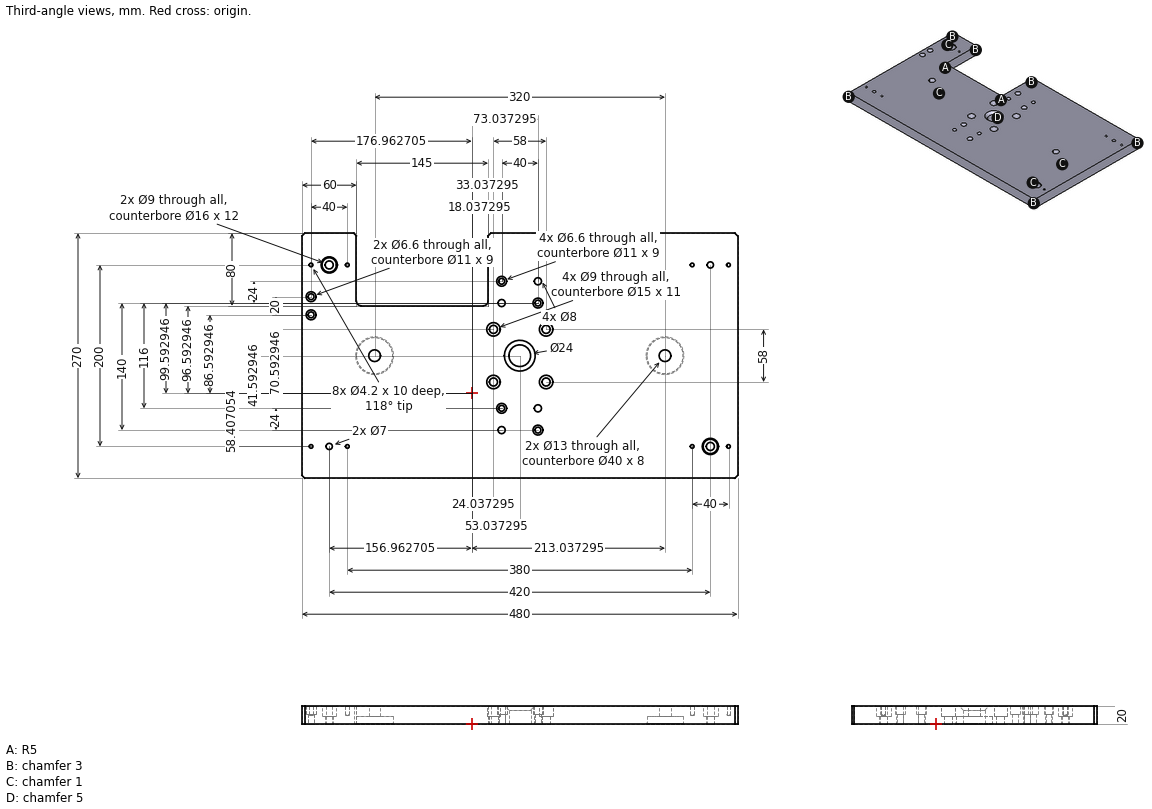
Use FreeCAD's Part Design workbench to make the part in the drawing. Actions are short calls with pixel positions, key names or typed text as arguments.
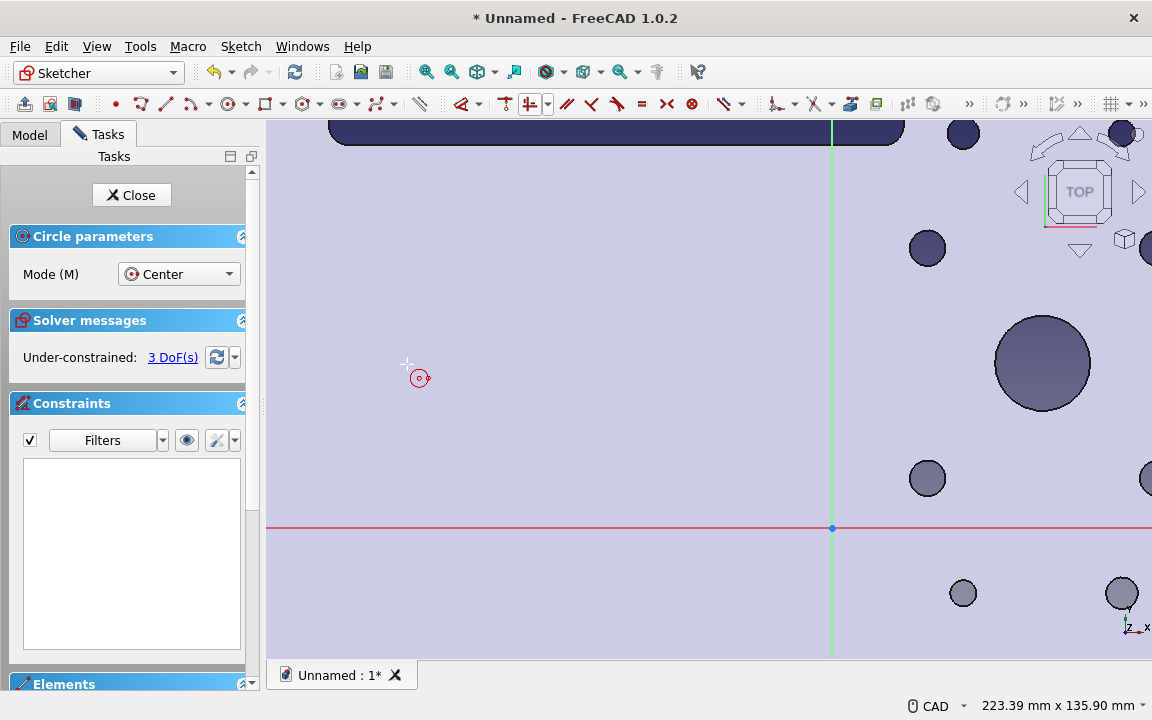
click(408, 363)
click(426, 345)
key(Escape)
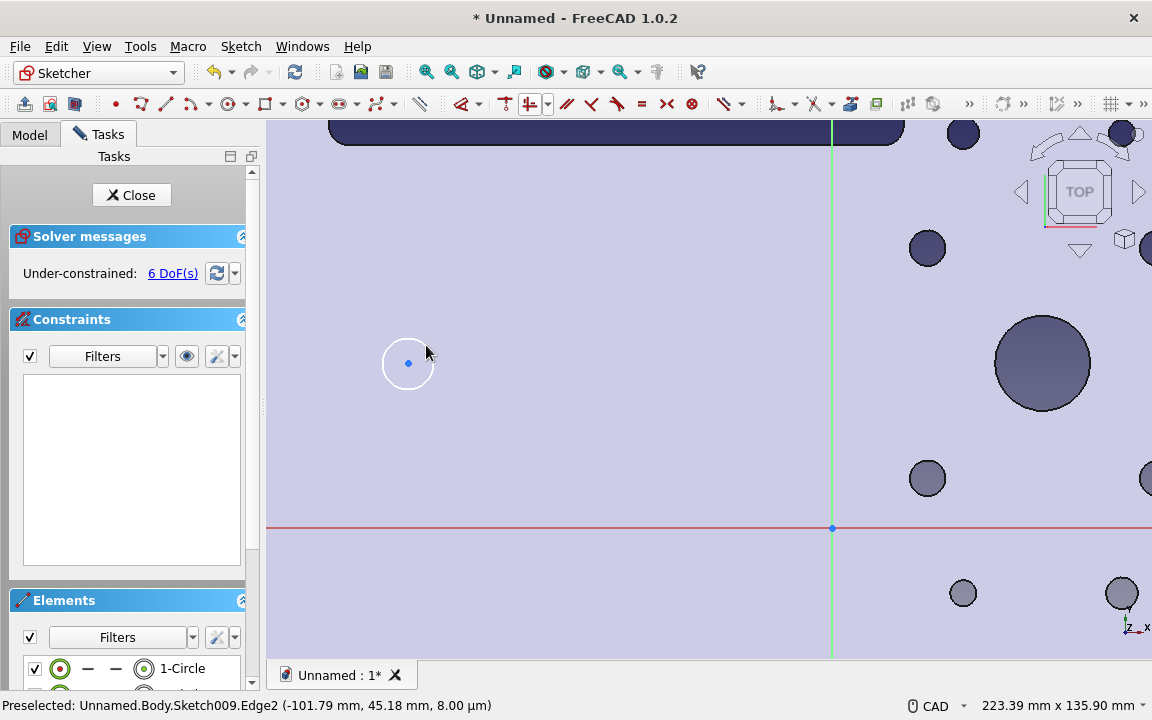
scroll(406, 364, down, 5)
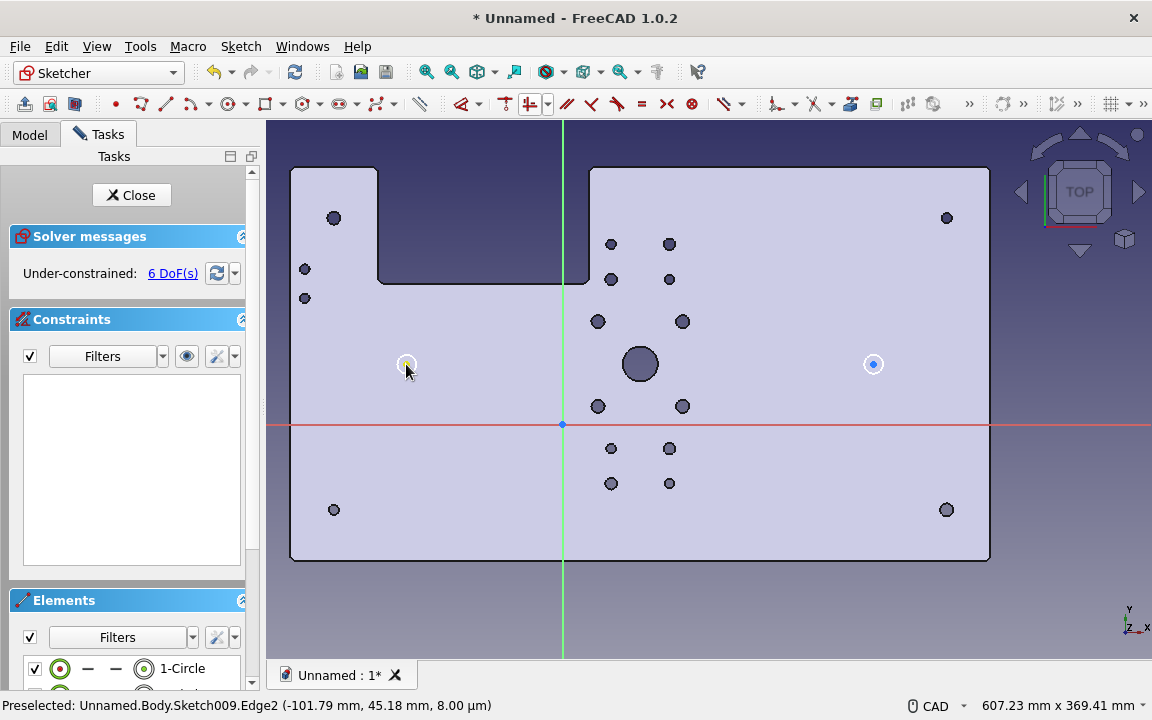
scroll(880, 358, up, 2)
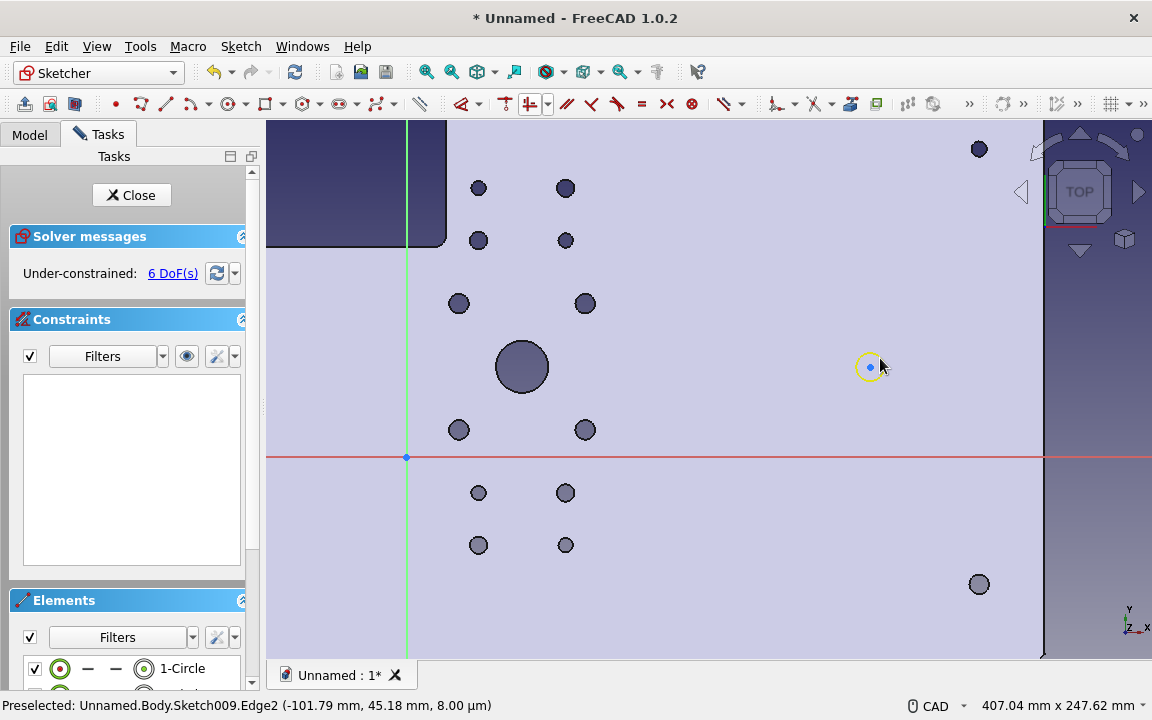
click(880, 357)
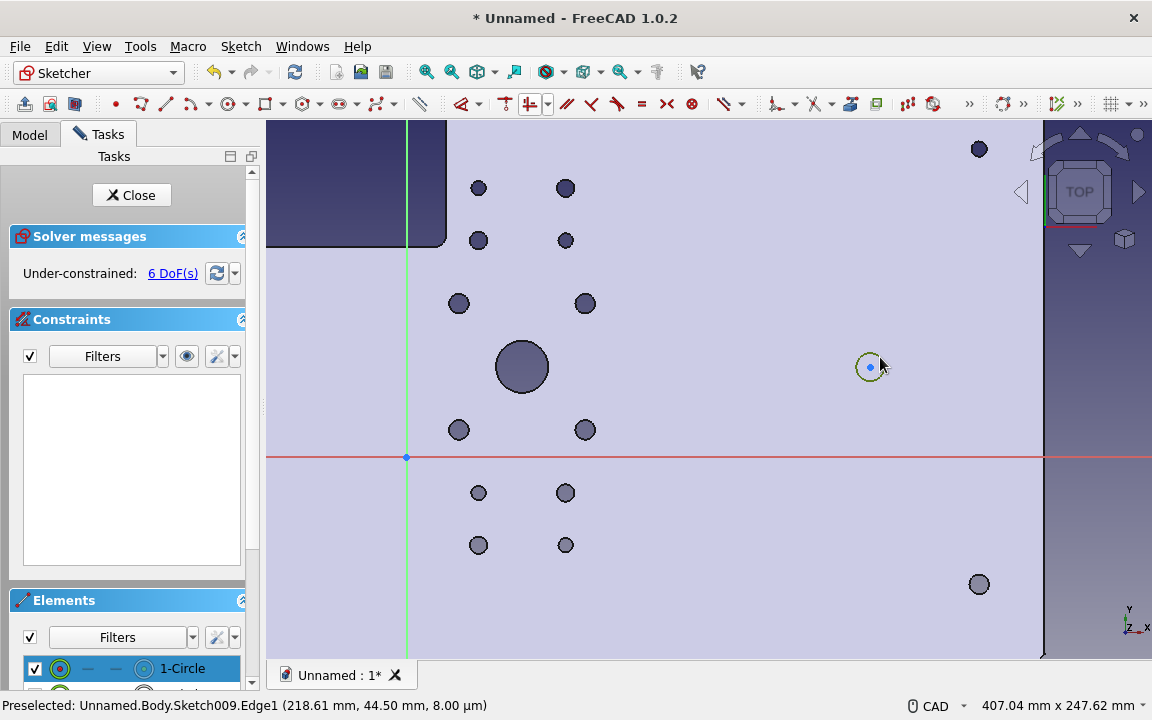
scroll(881, 358, down, 2)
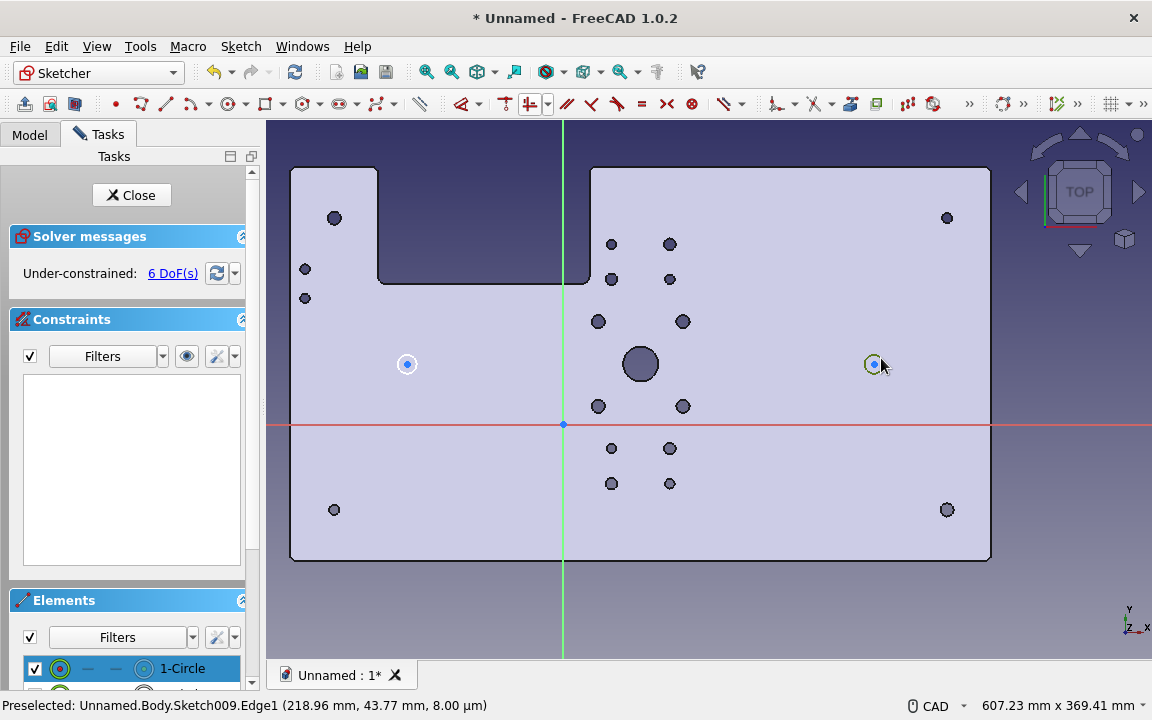
scroll(414, 358, up, 2)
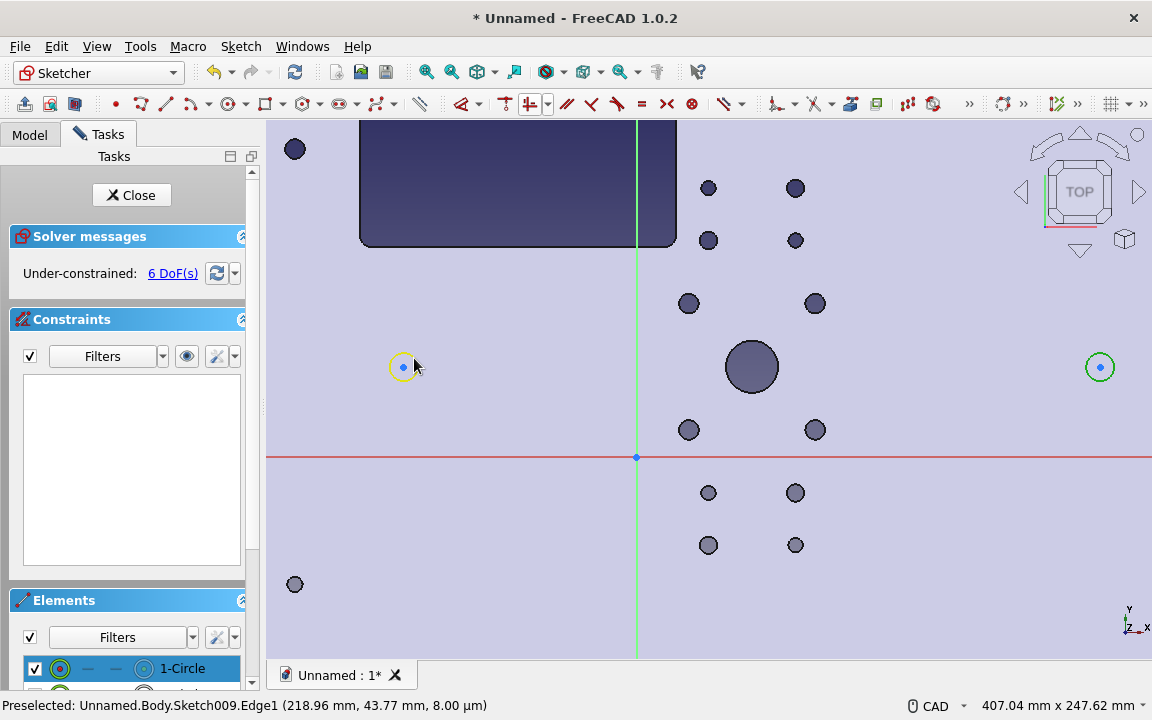
click(414, 357)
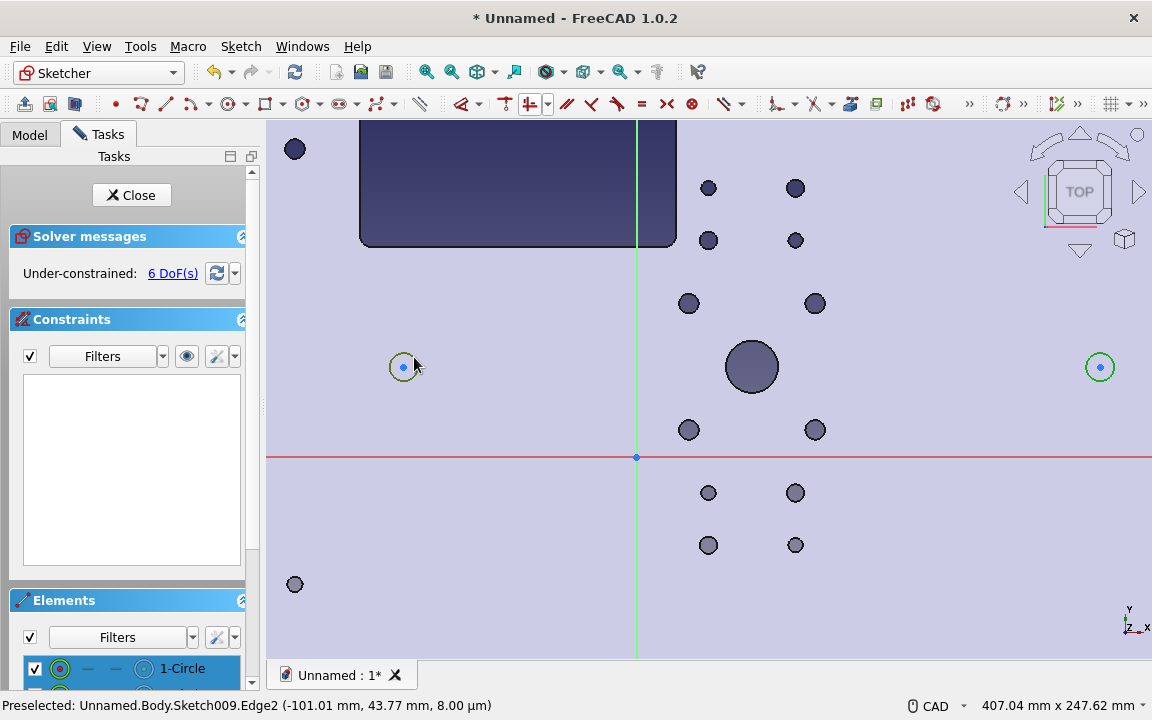
key(e)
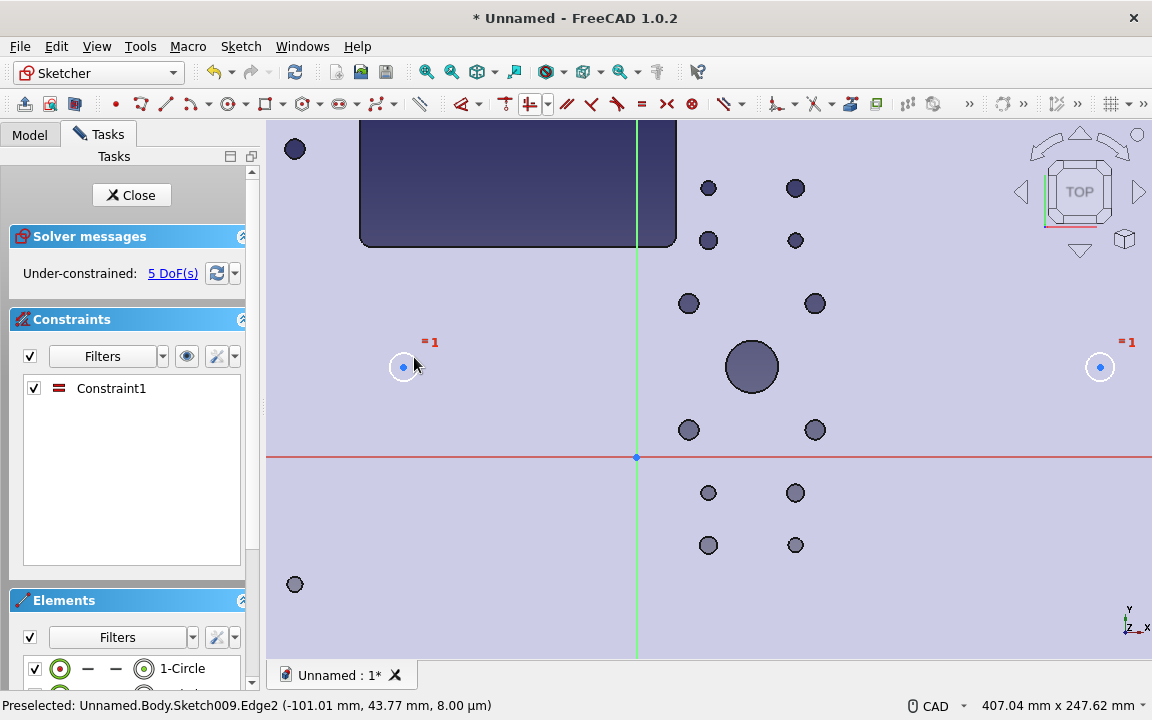
scroll(414, 358, down, 2)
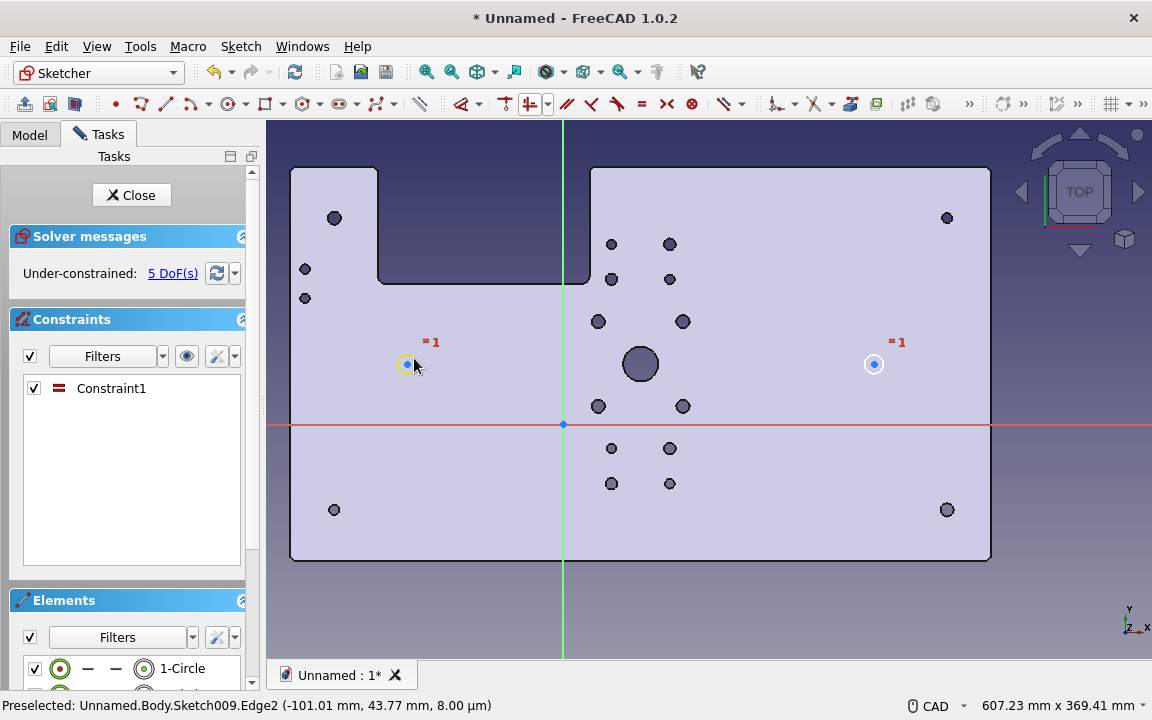
click(874, 364)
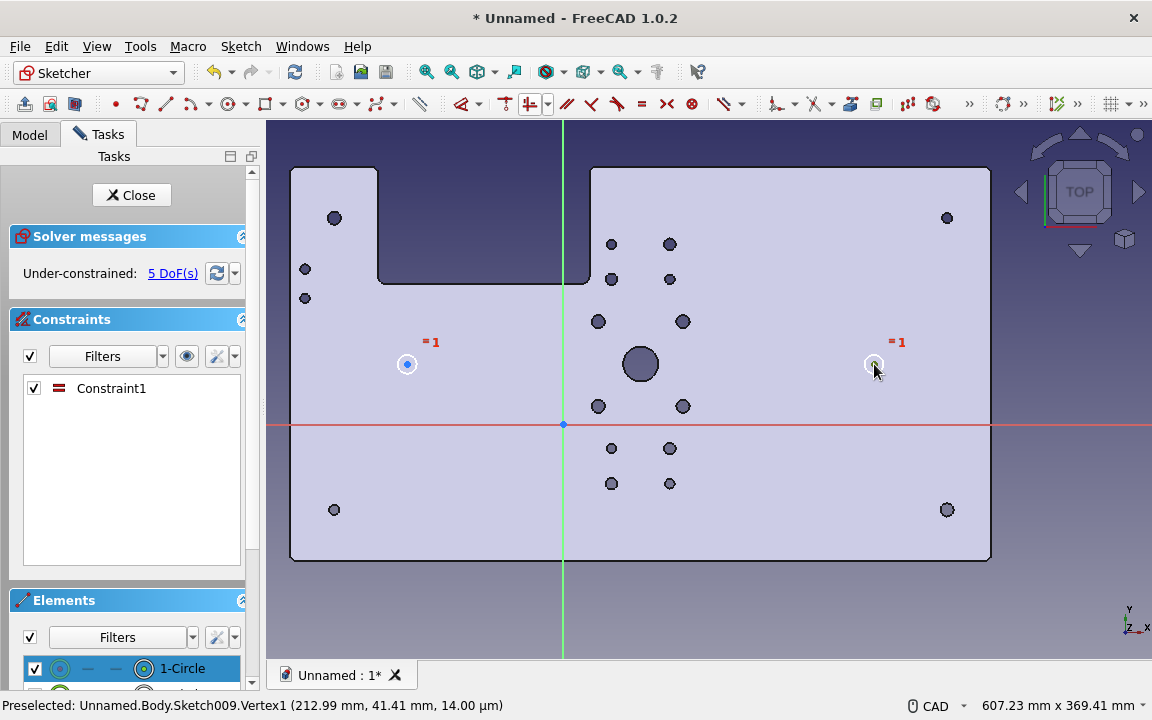
click(407, 364)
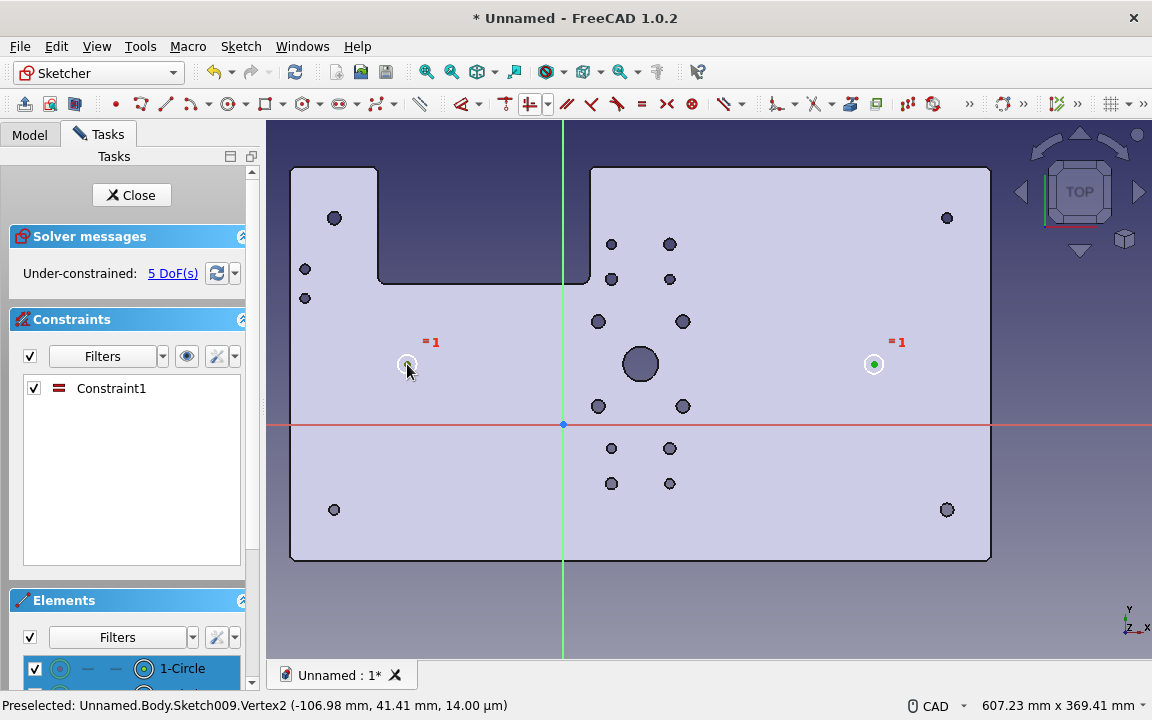
click(548, 104)